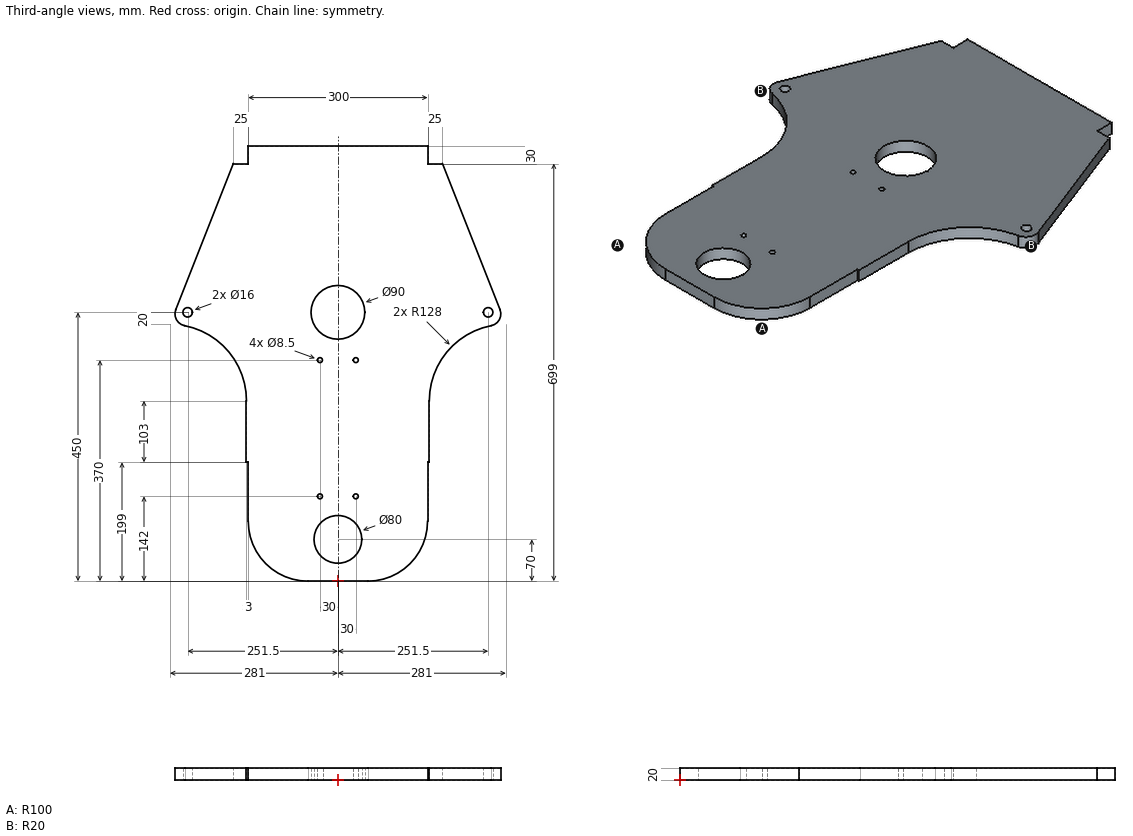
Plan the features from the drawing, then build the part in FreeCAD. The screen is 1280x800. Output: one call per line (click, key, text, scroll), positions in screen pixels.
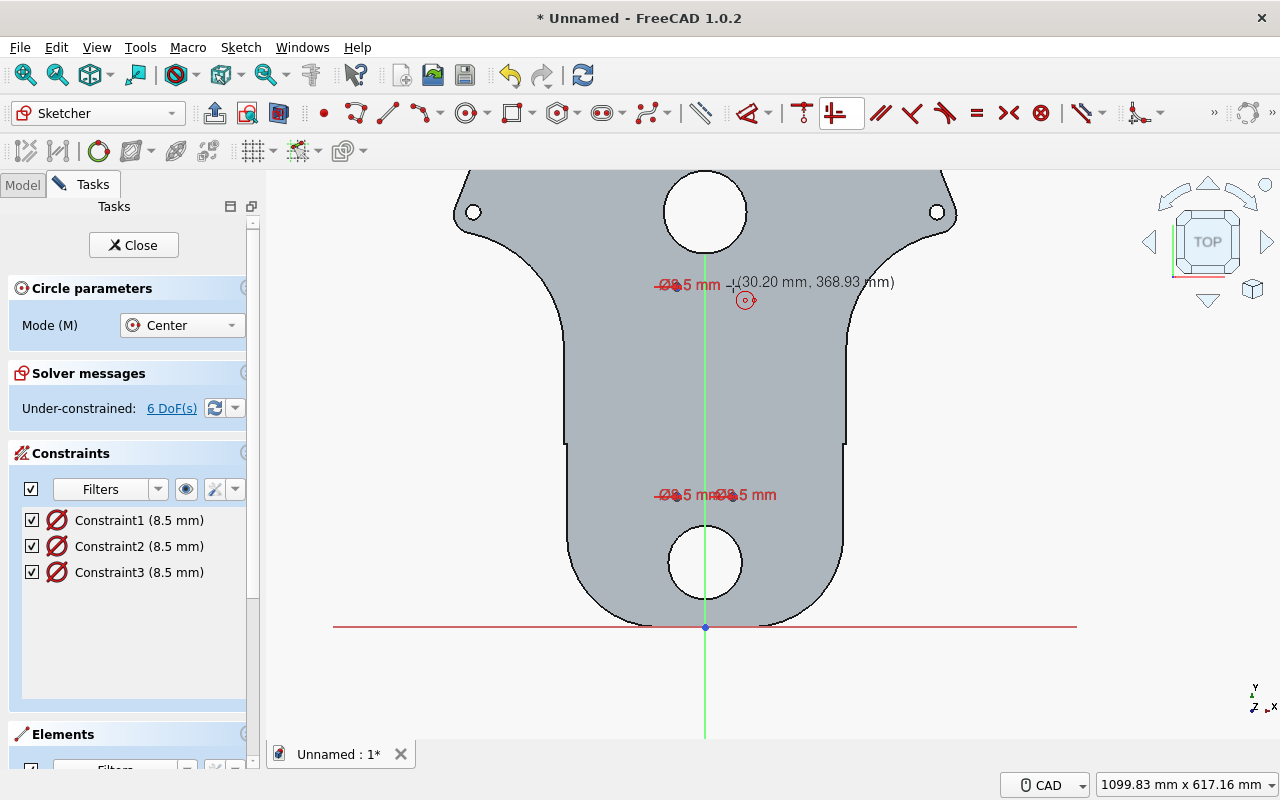
click(733, 286)
move(736, 283)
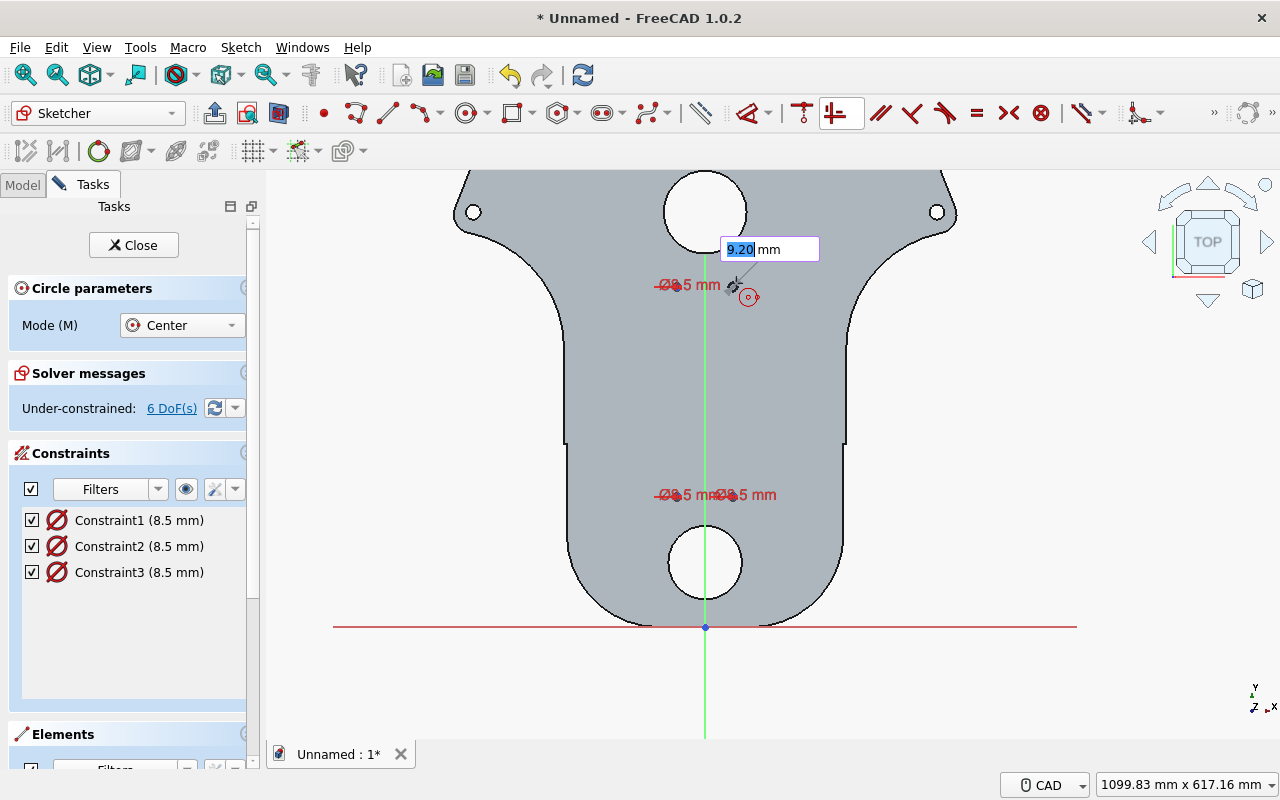
text(8.5)
key(Return)
key(Escape)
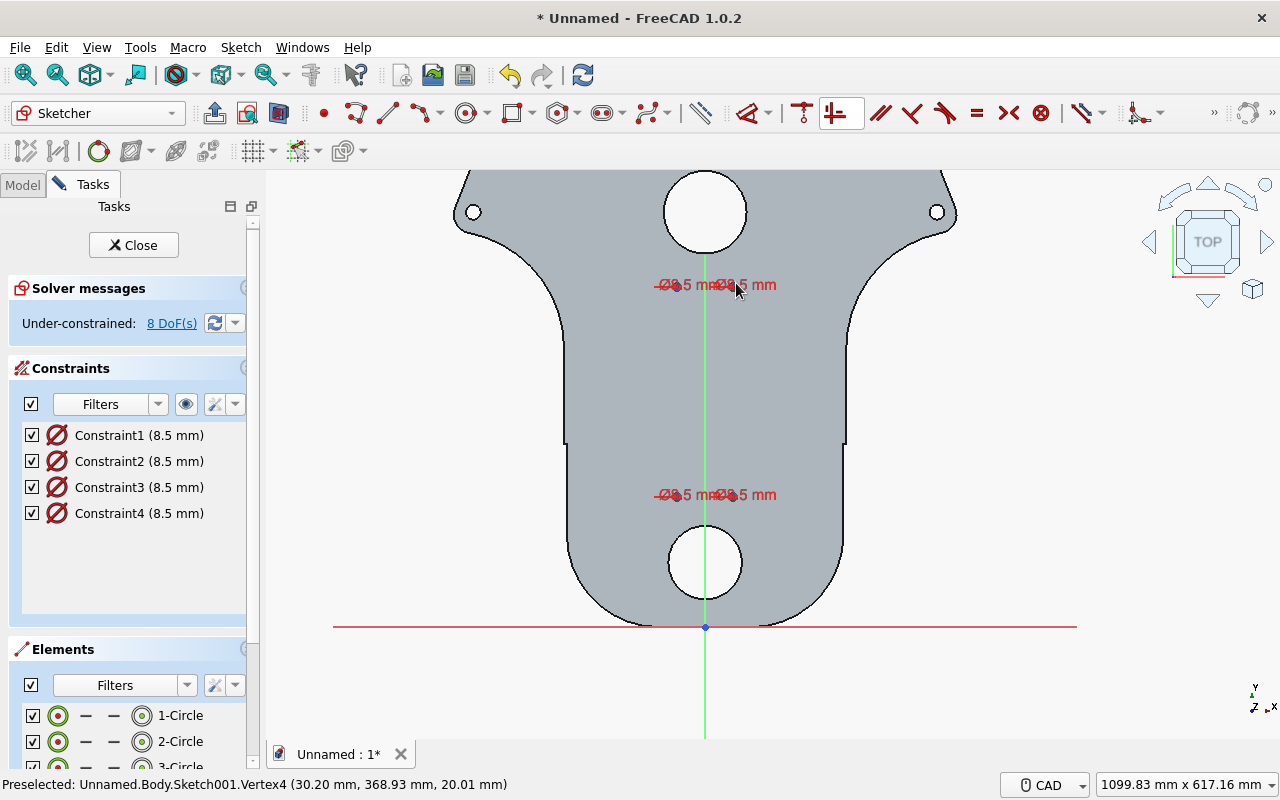
click(677, 287)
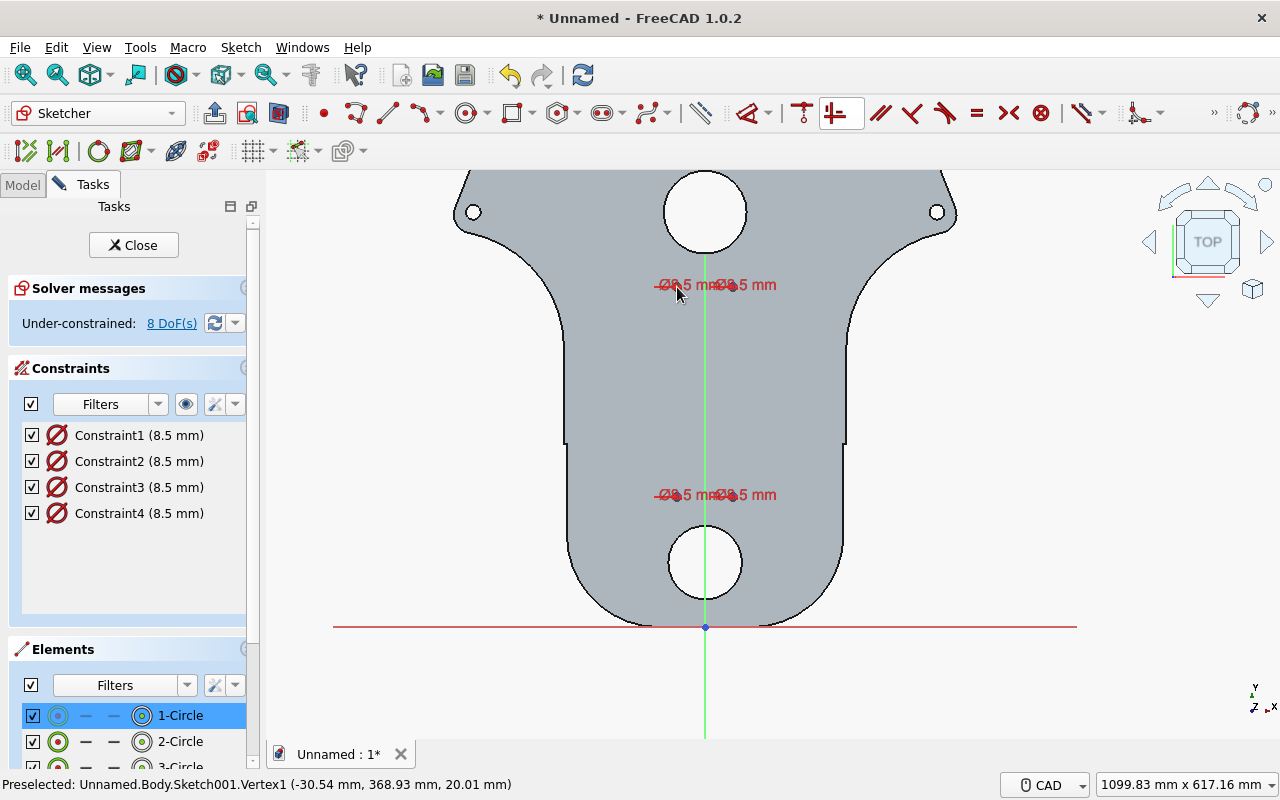
click(677, 497)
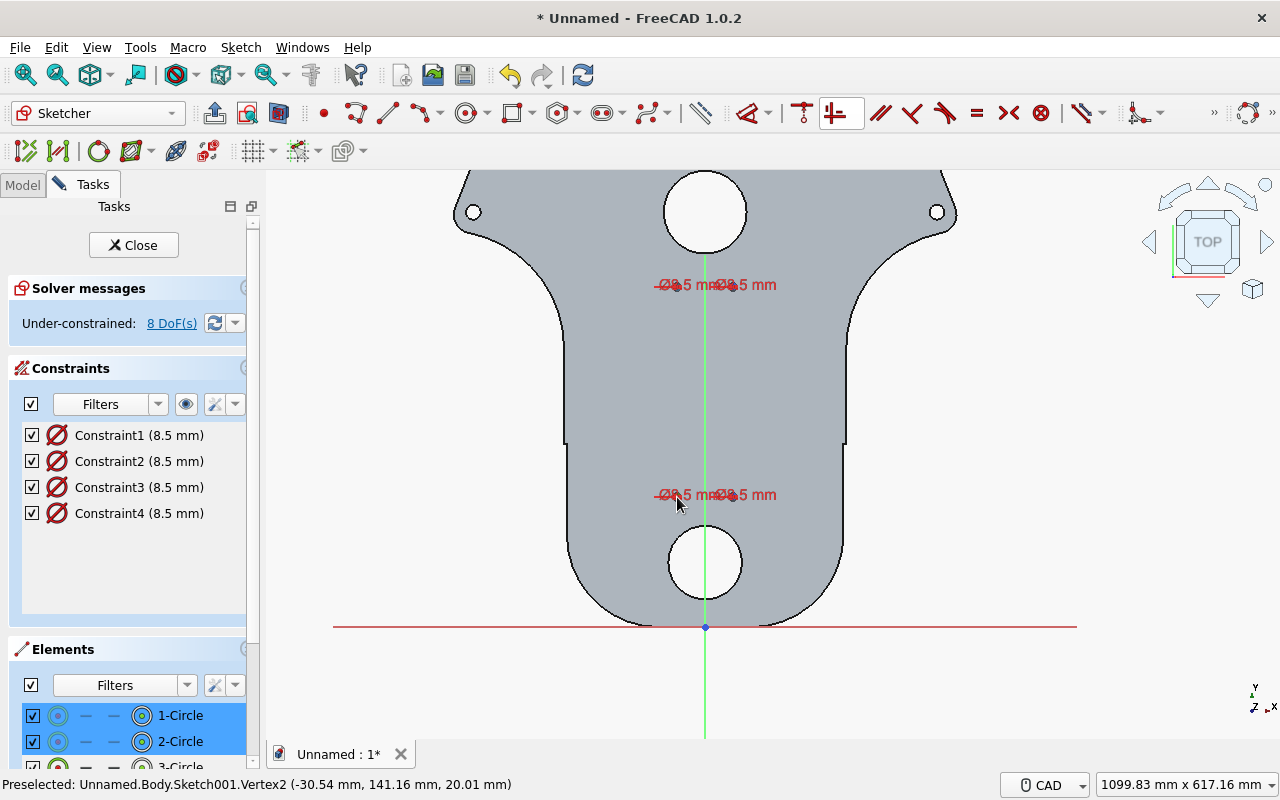
key(v)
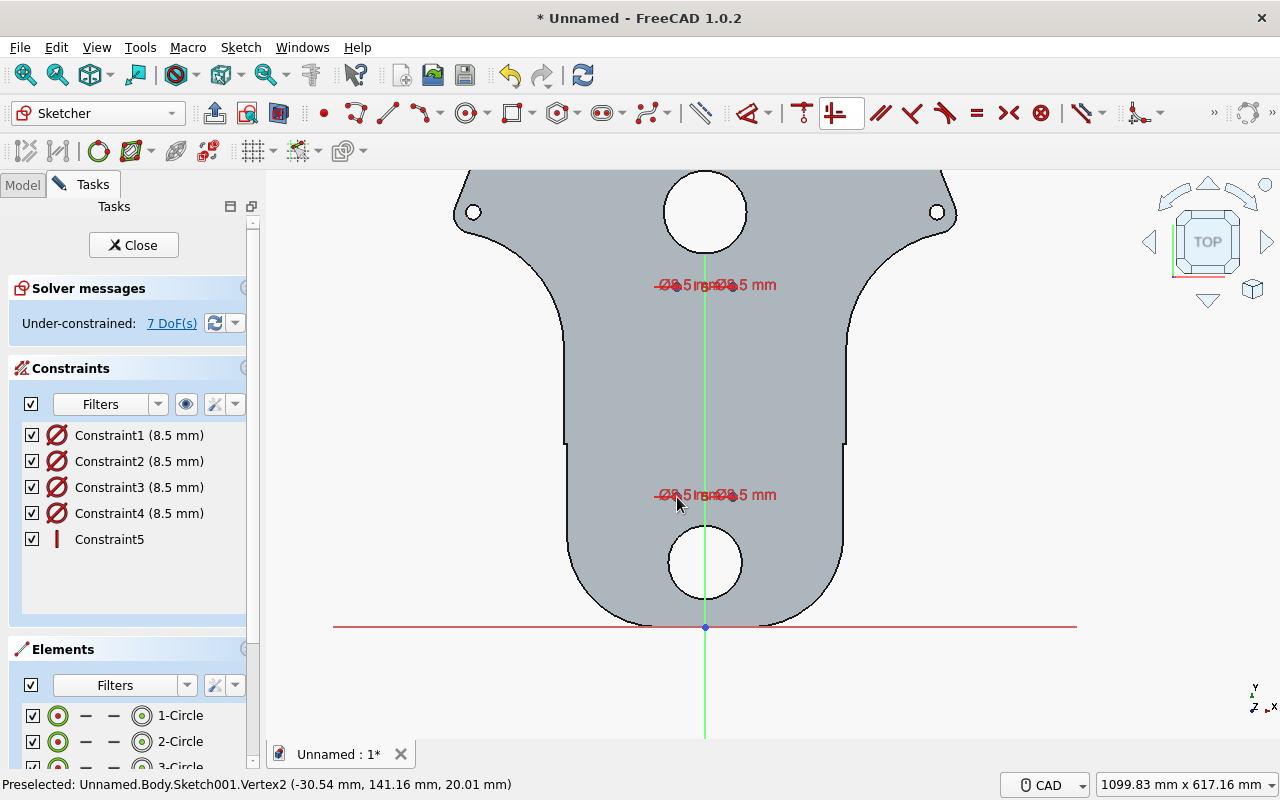
click(677, 497)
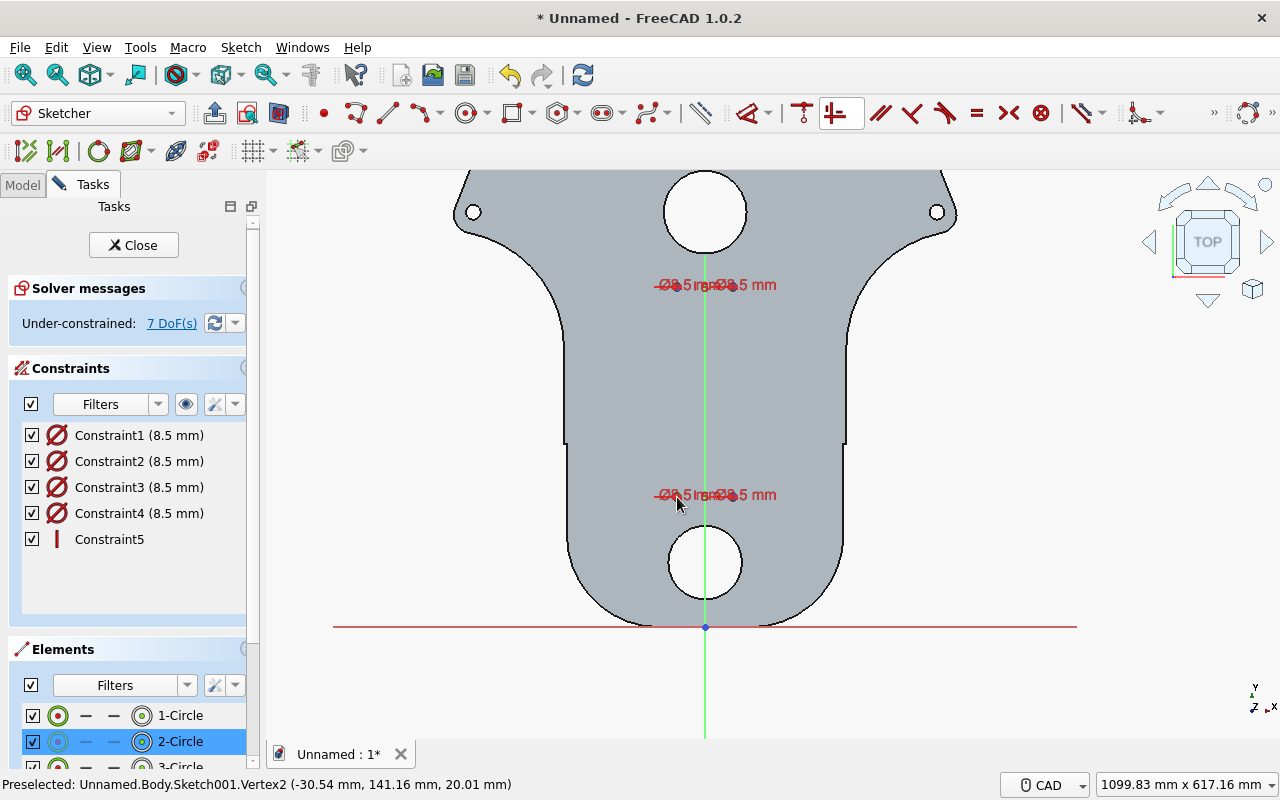
click(733, 497)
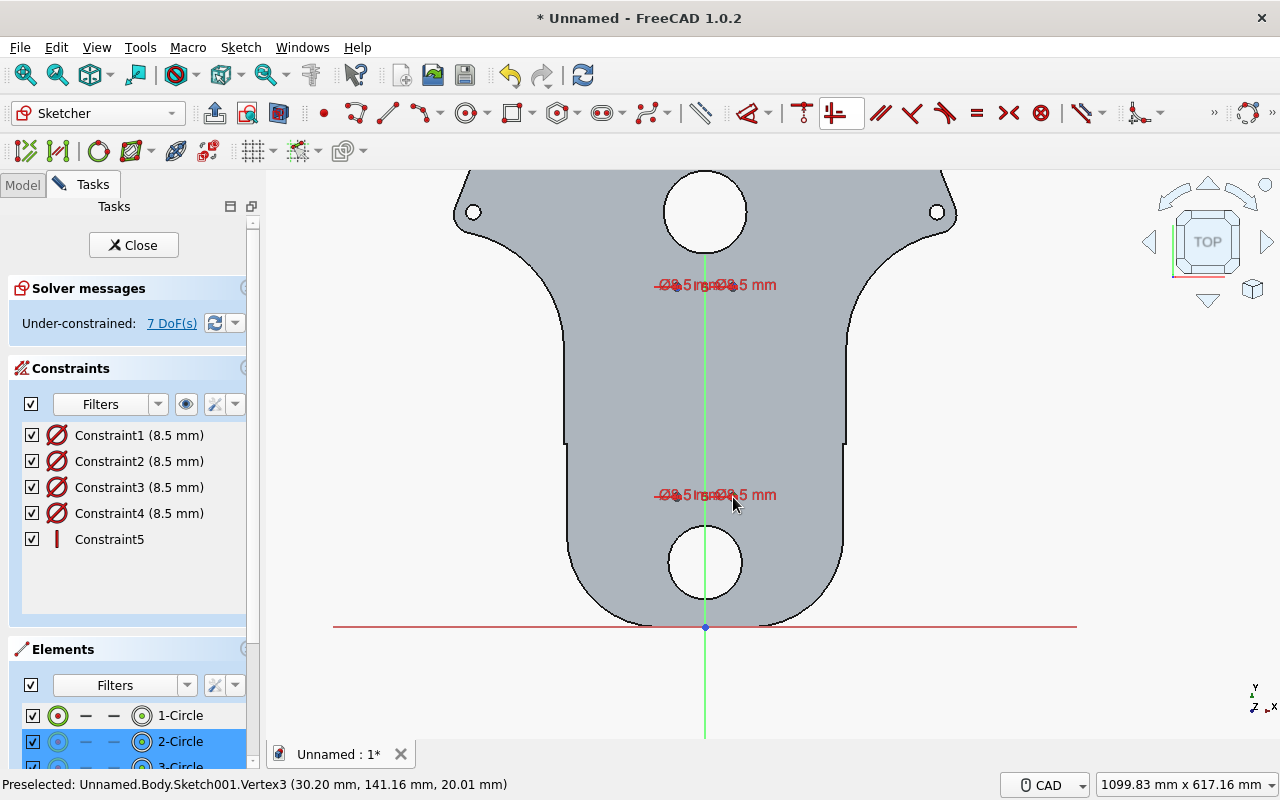
click(858, 114)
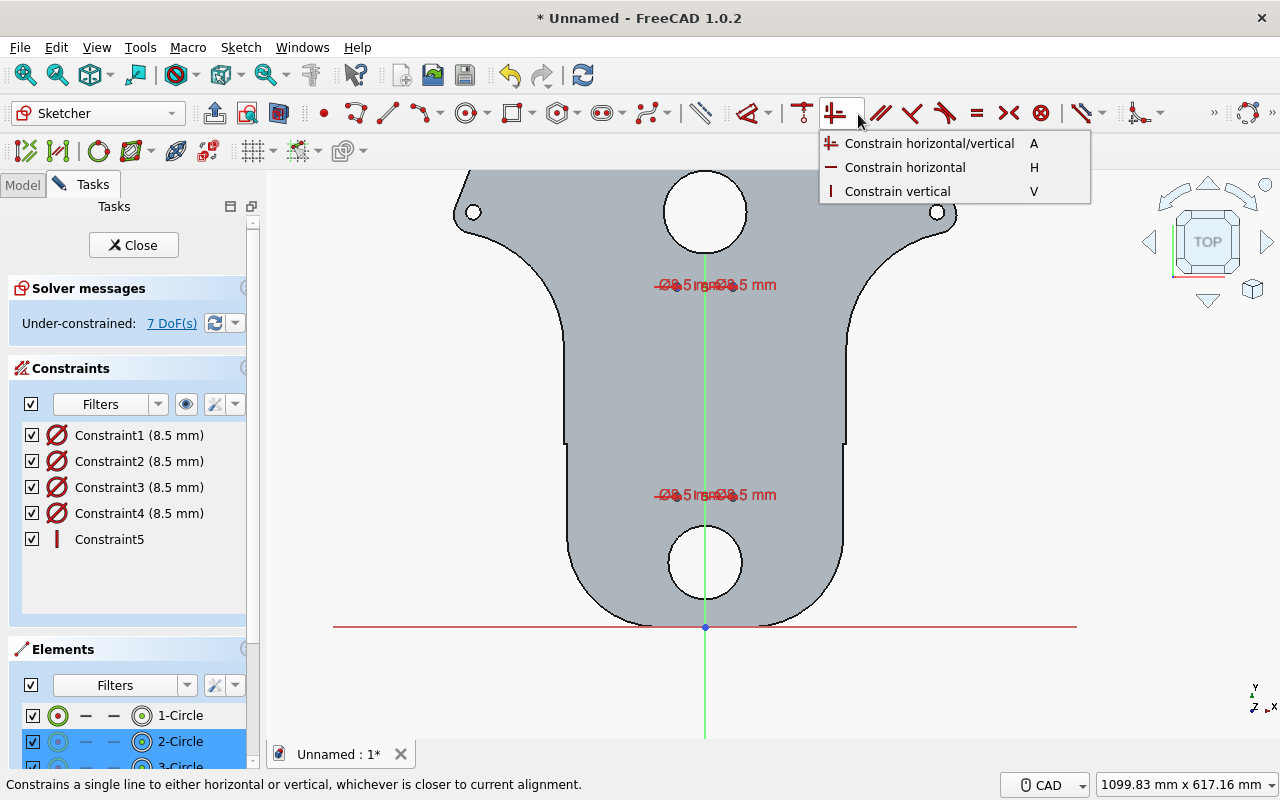
click(955, 167)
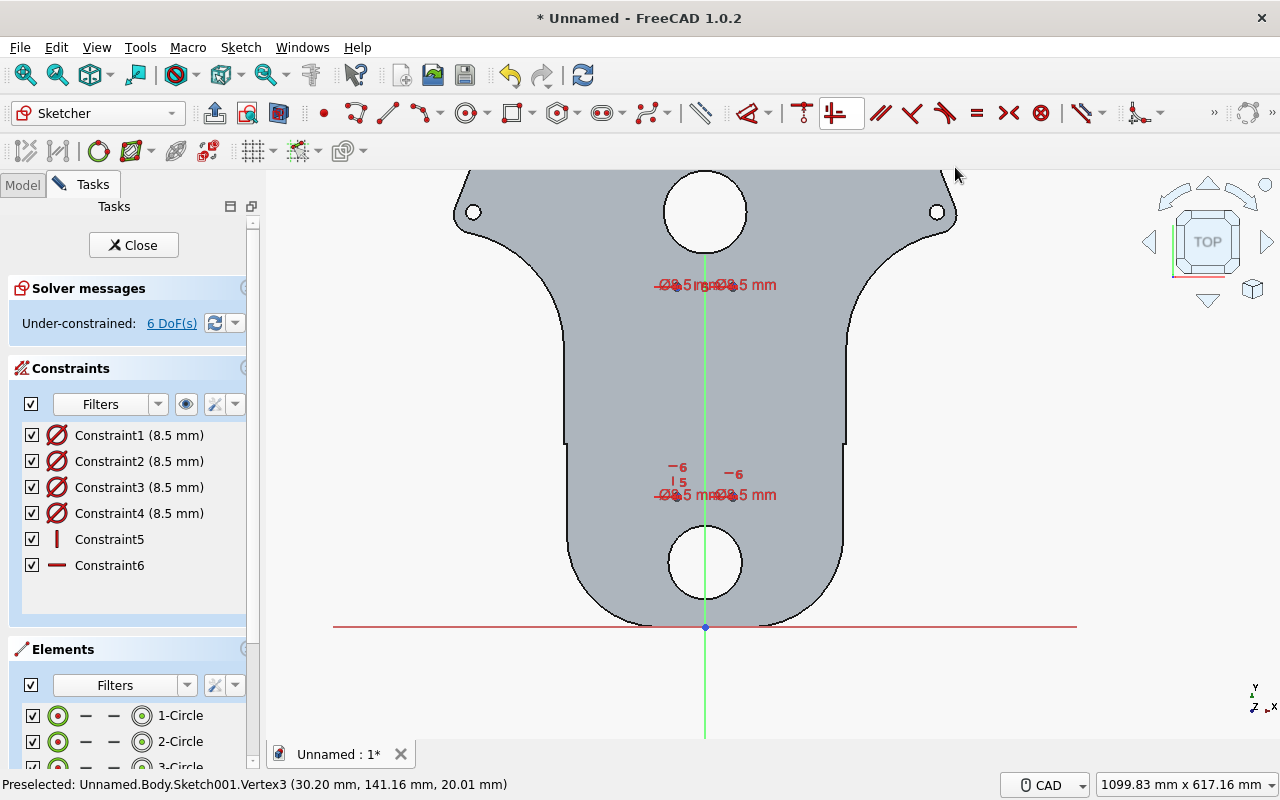
click(733, 497)